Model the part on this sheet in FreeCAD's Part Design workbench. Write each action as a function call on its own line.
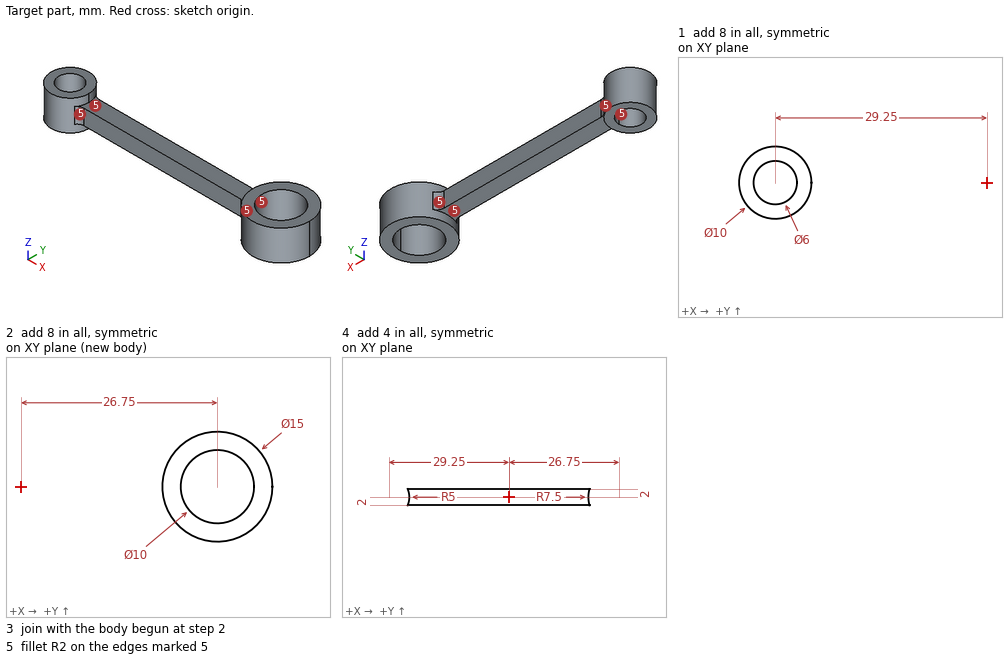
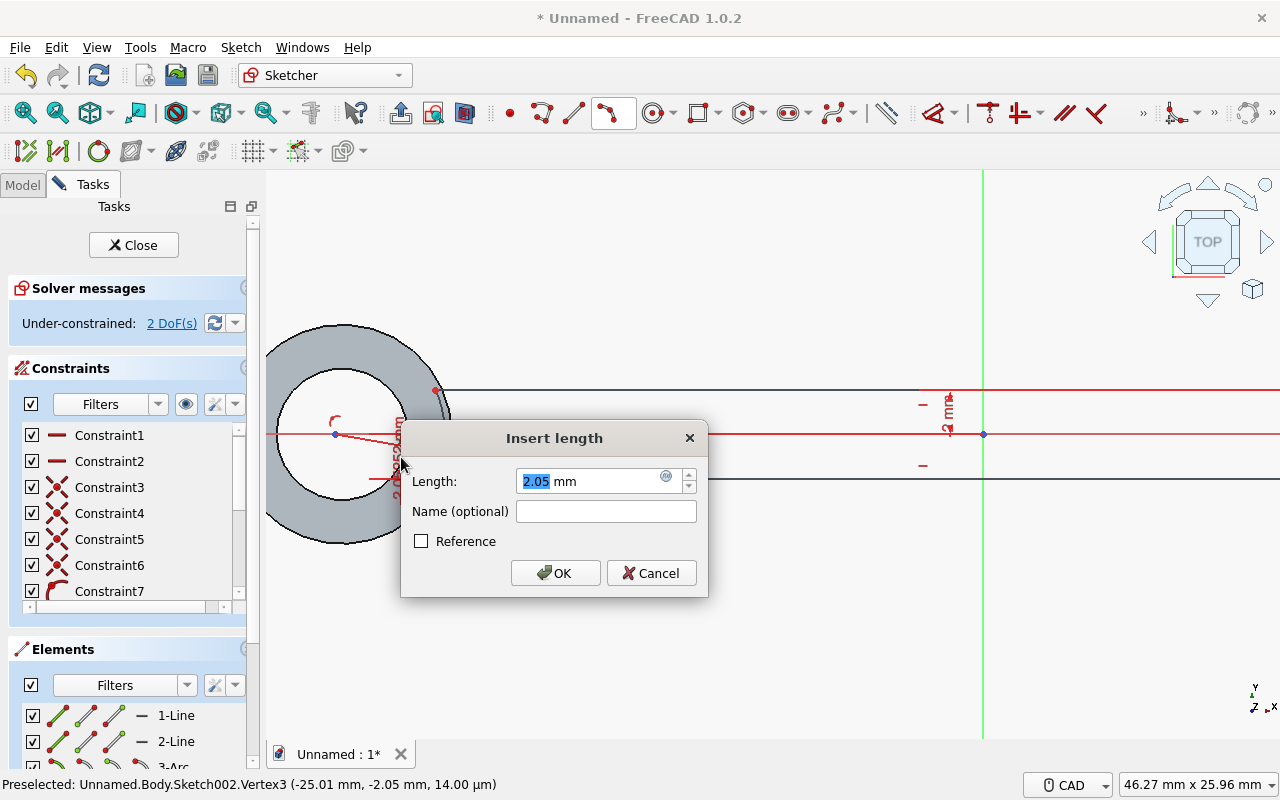
text(2)
key(Return)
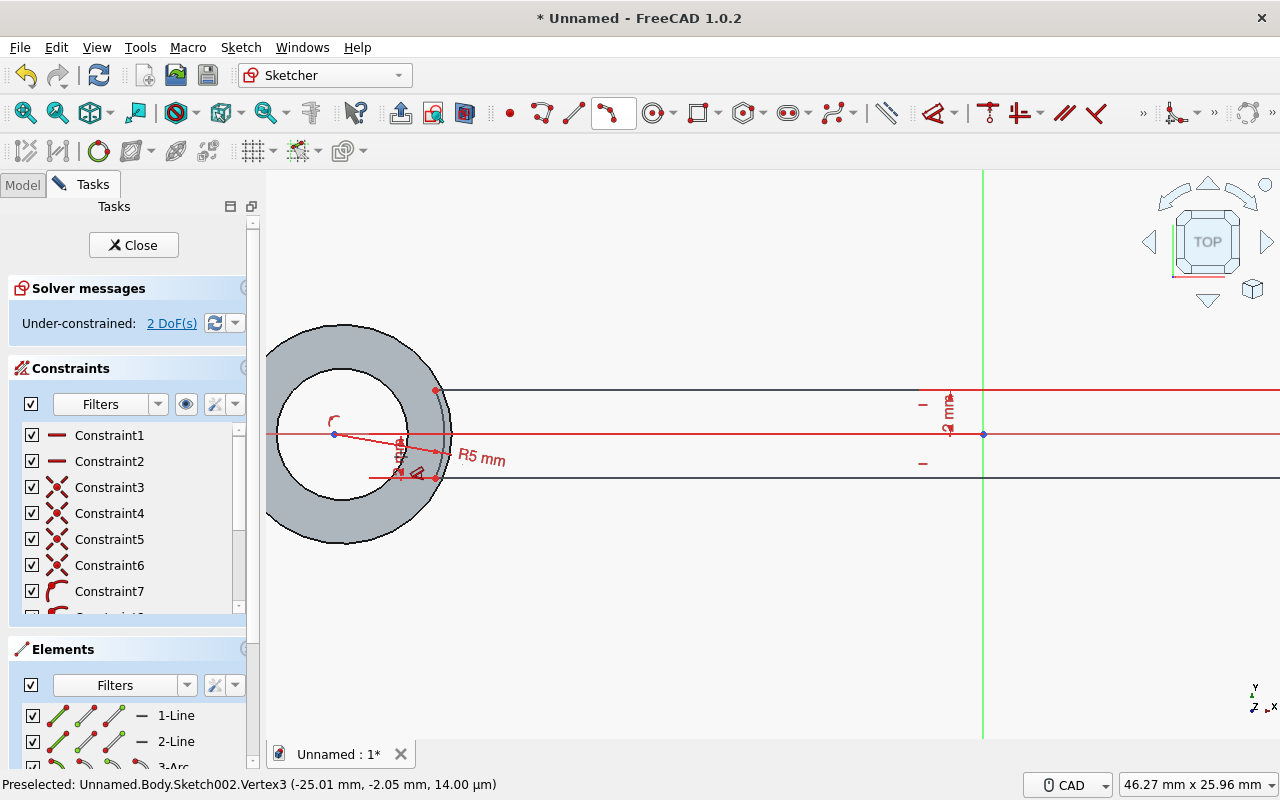
click(335, 434)
click(659, 492)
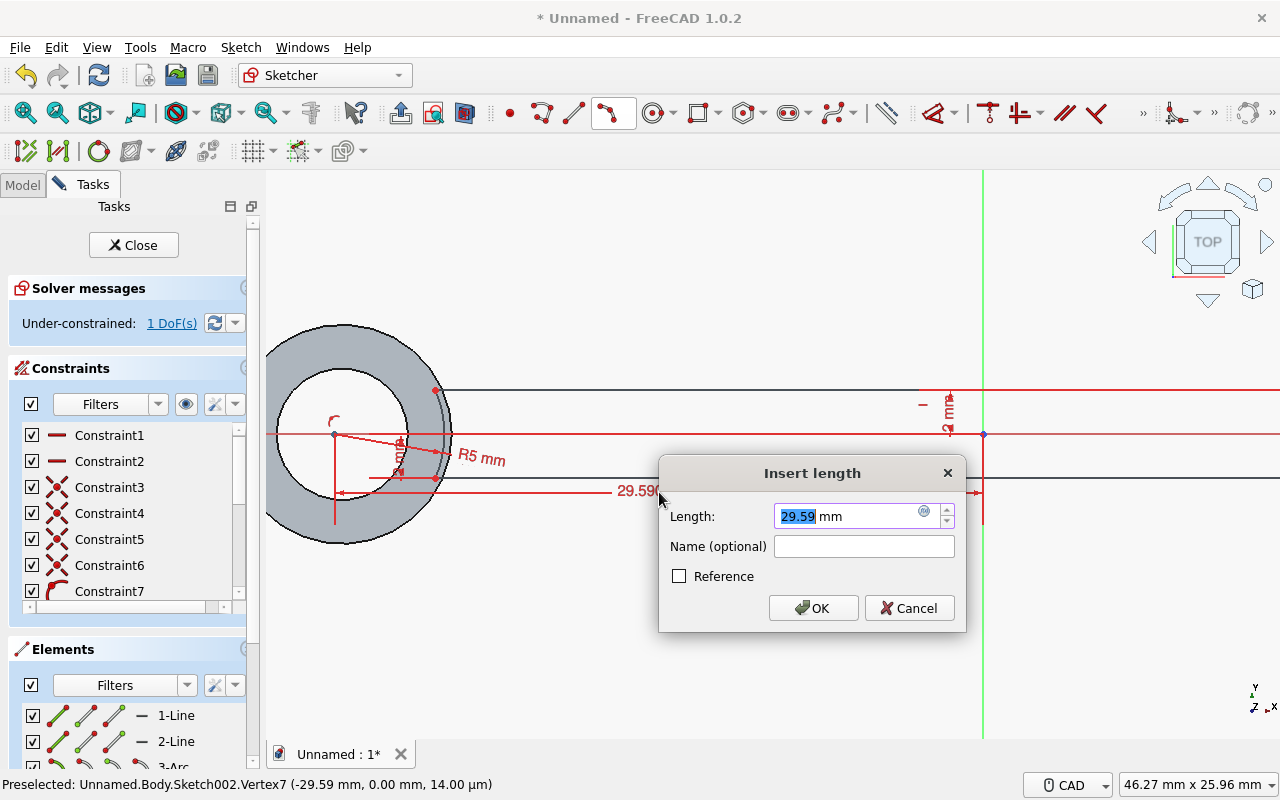
text(29.25)
key(Return)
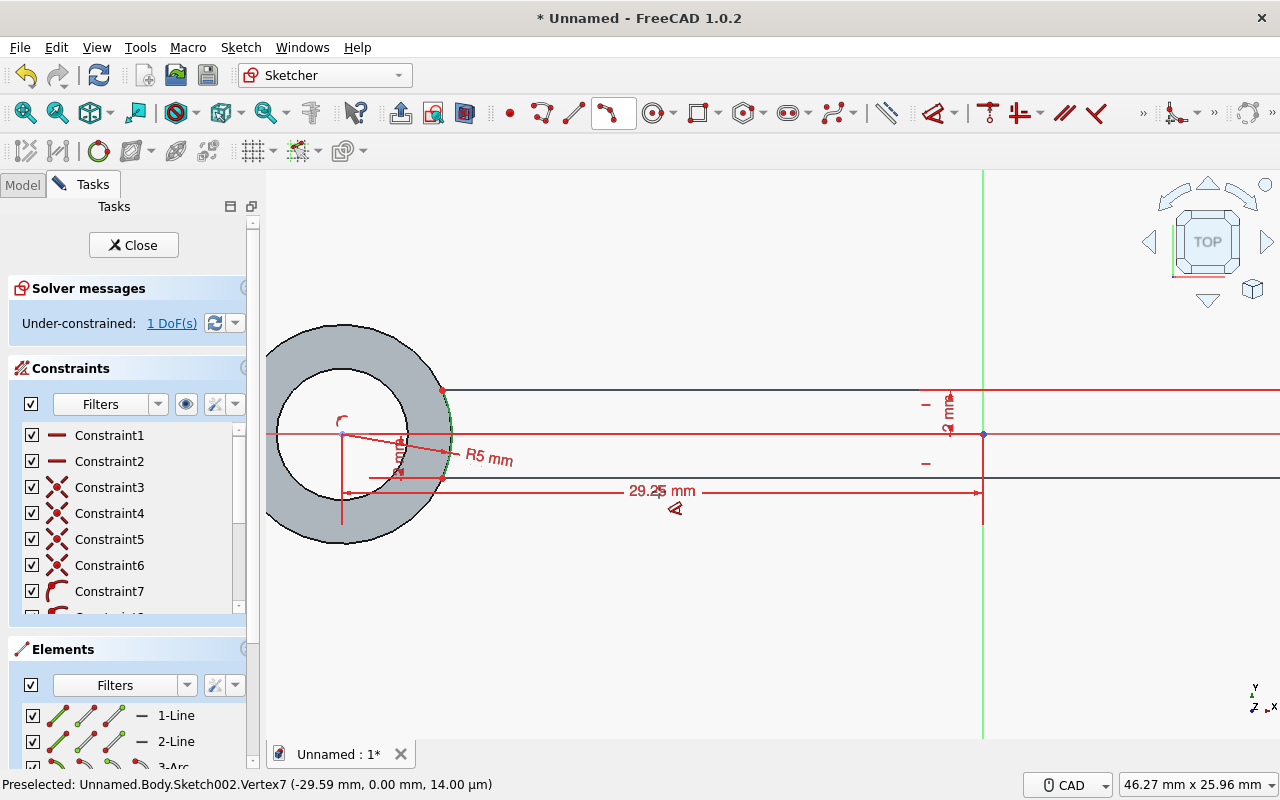
scroll(434, 479, down, 3)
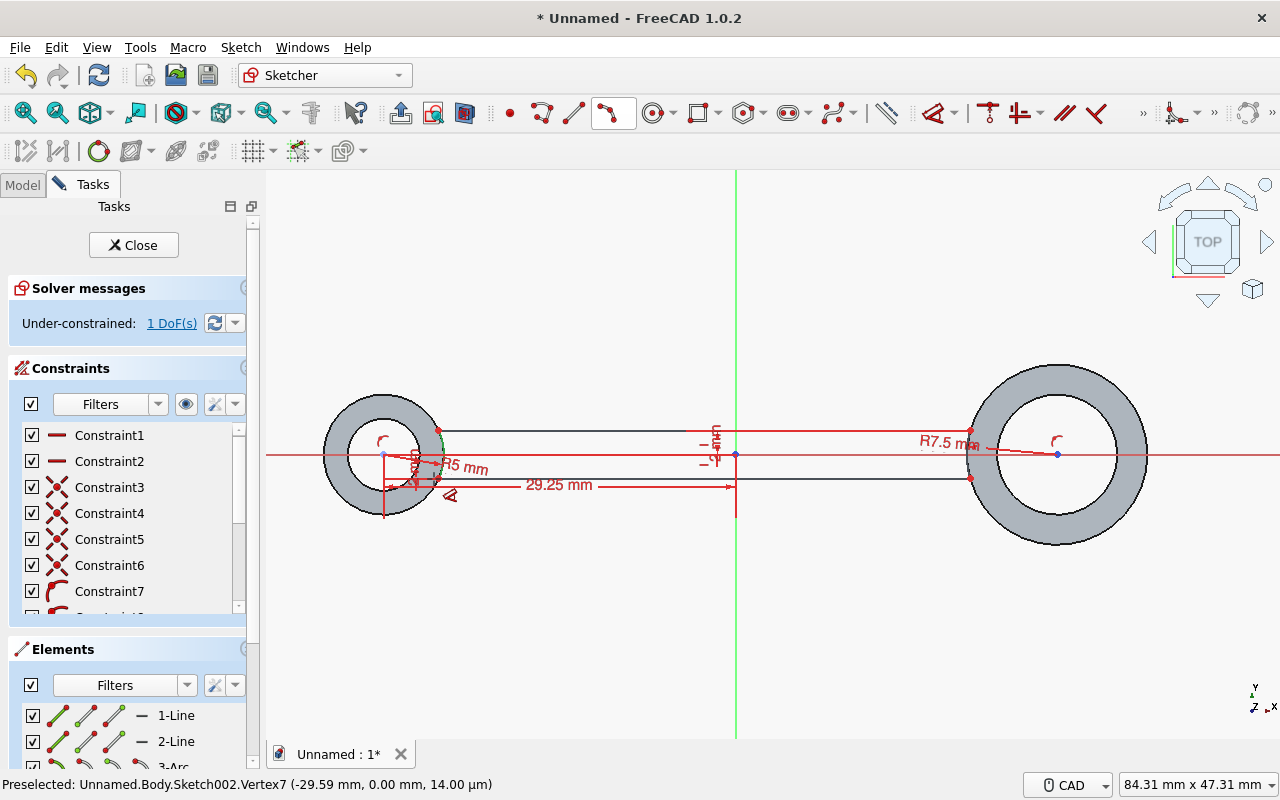
click(1057, 455)
click(1009, 489)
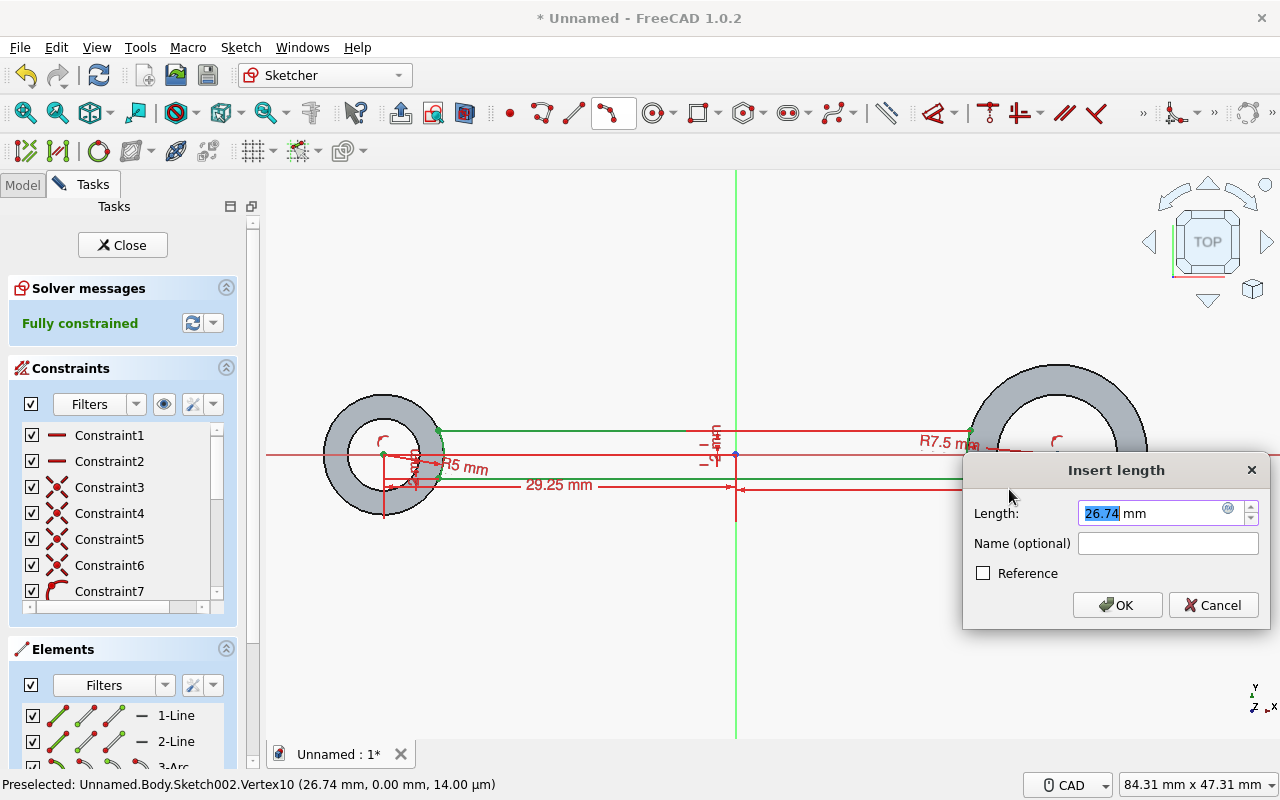
text(26.75)
key(Return)
key(Escape)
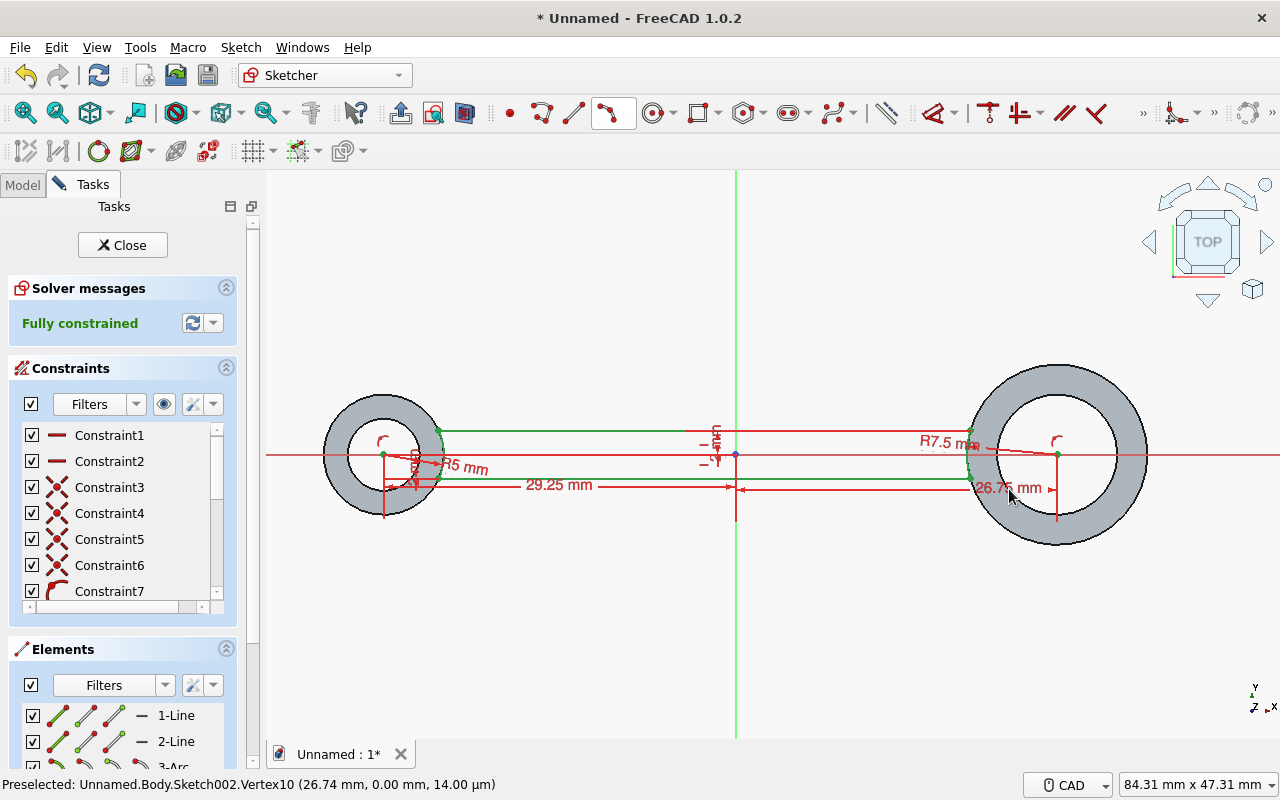
click(123, 245)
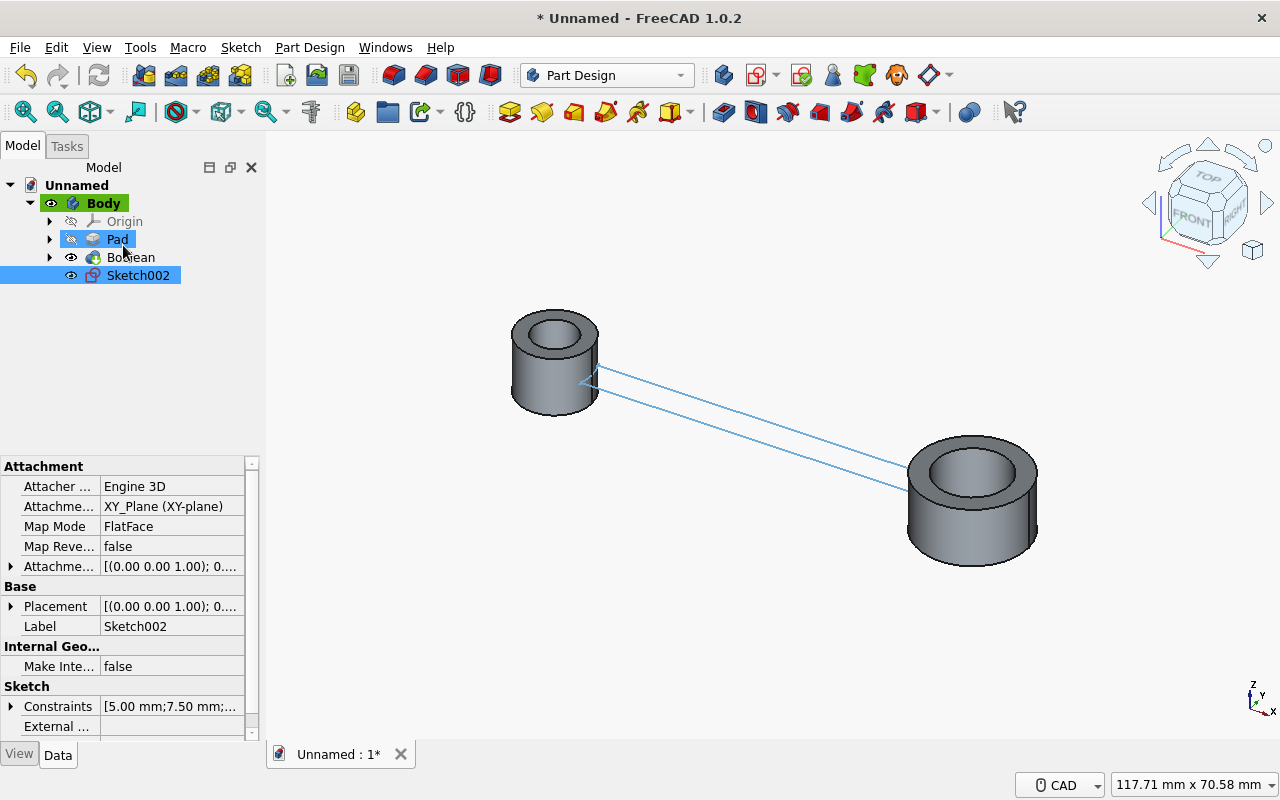
click(510, 112)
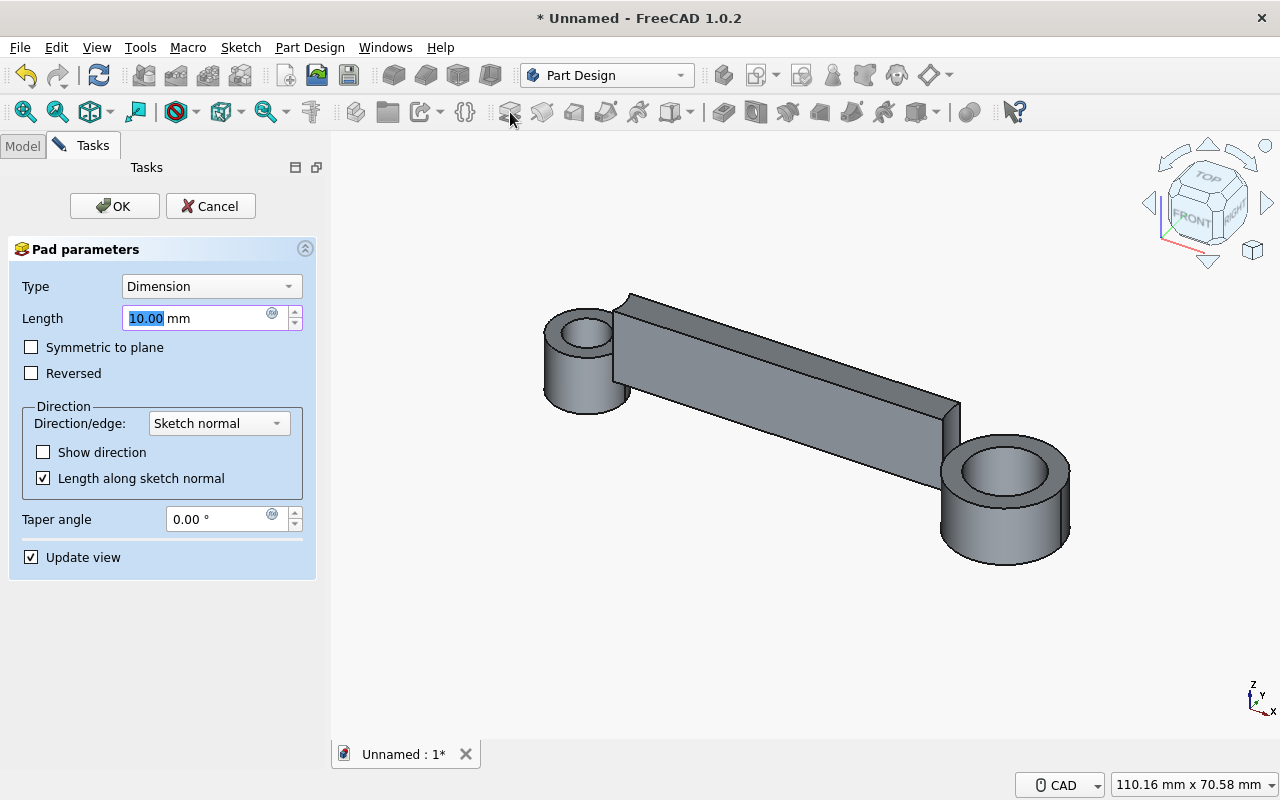
text(4)
key(Tab)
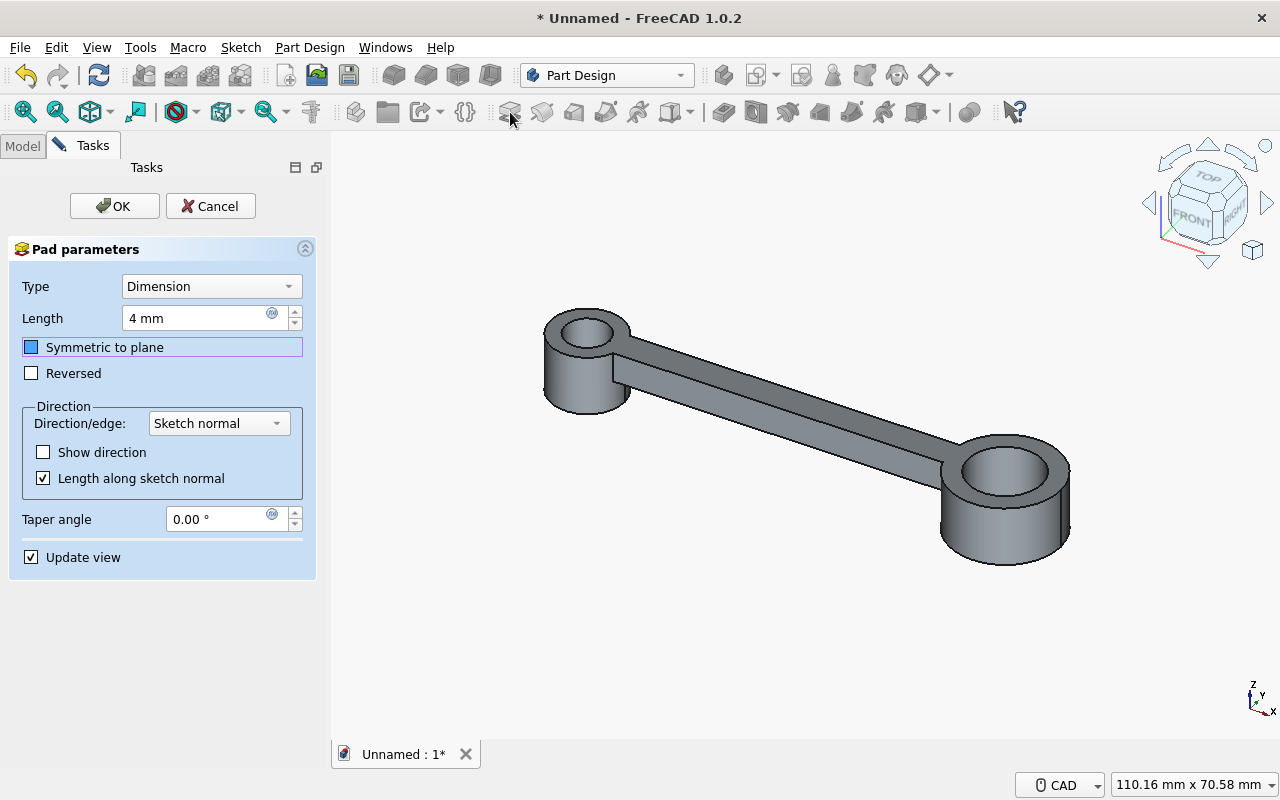
click(30, 347)